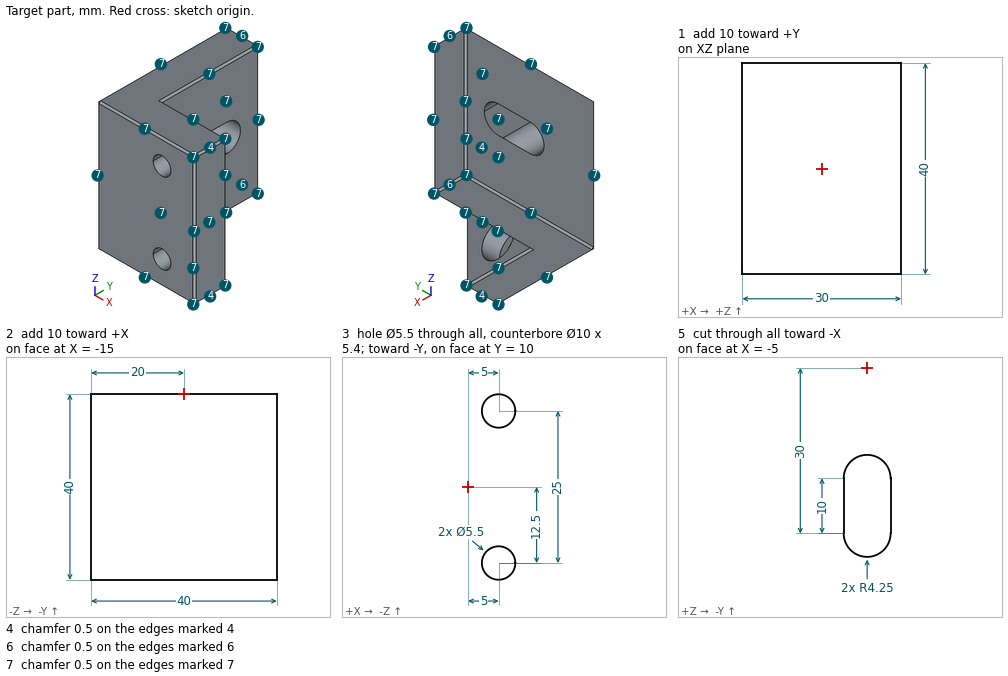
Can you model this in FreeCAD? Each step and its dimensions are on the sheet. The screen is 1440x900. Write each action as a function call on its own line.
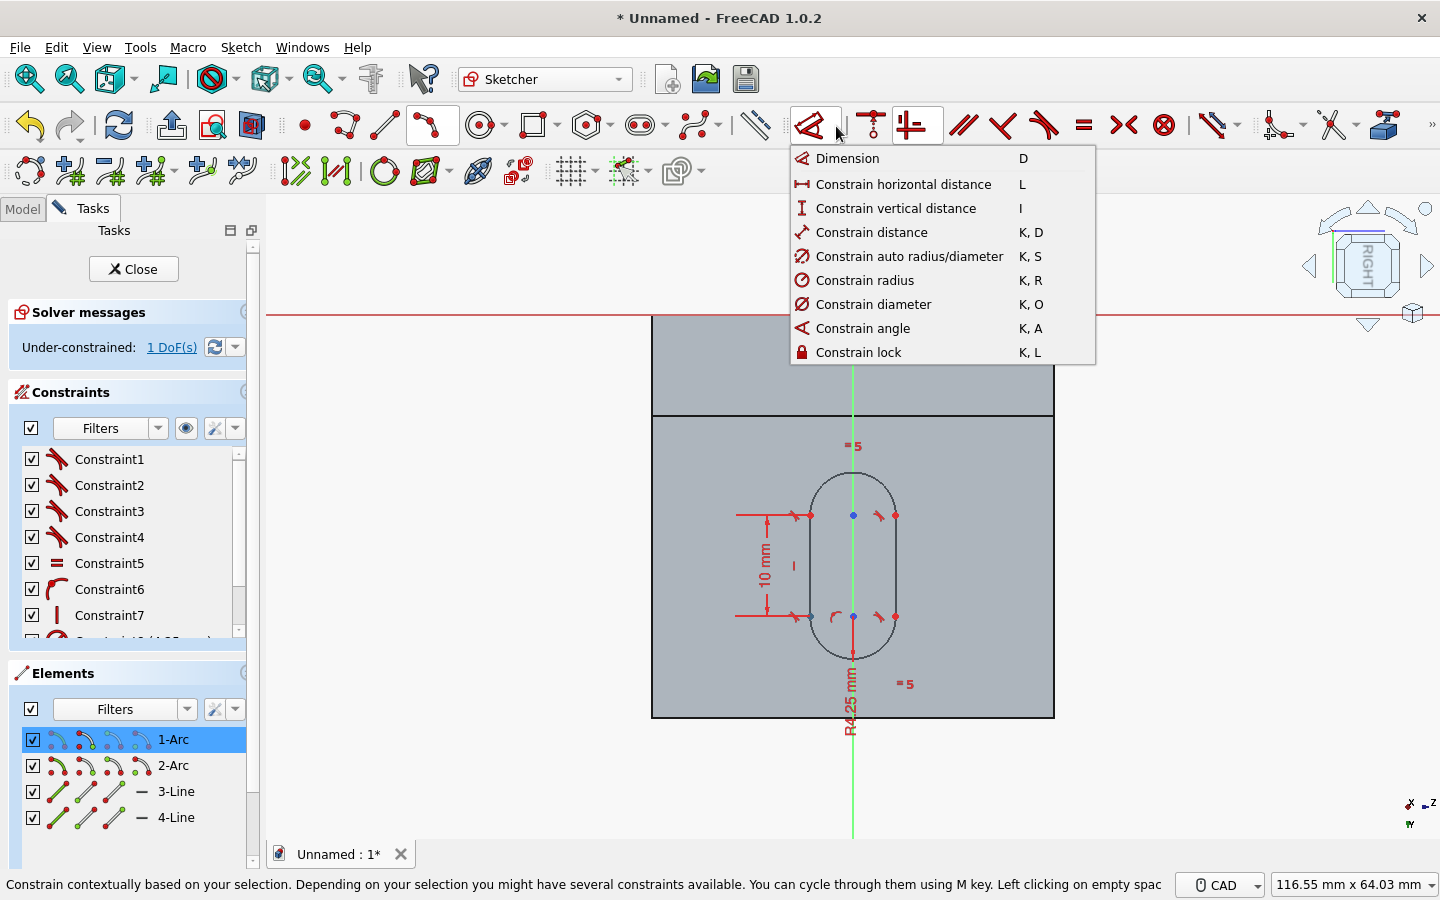
click(943, 208)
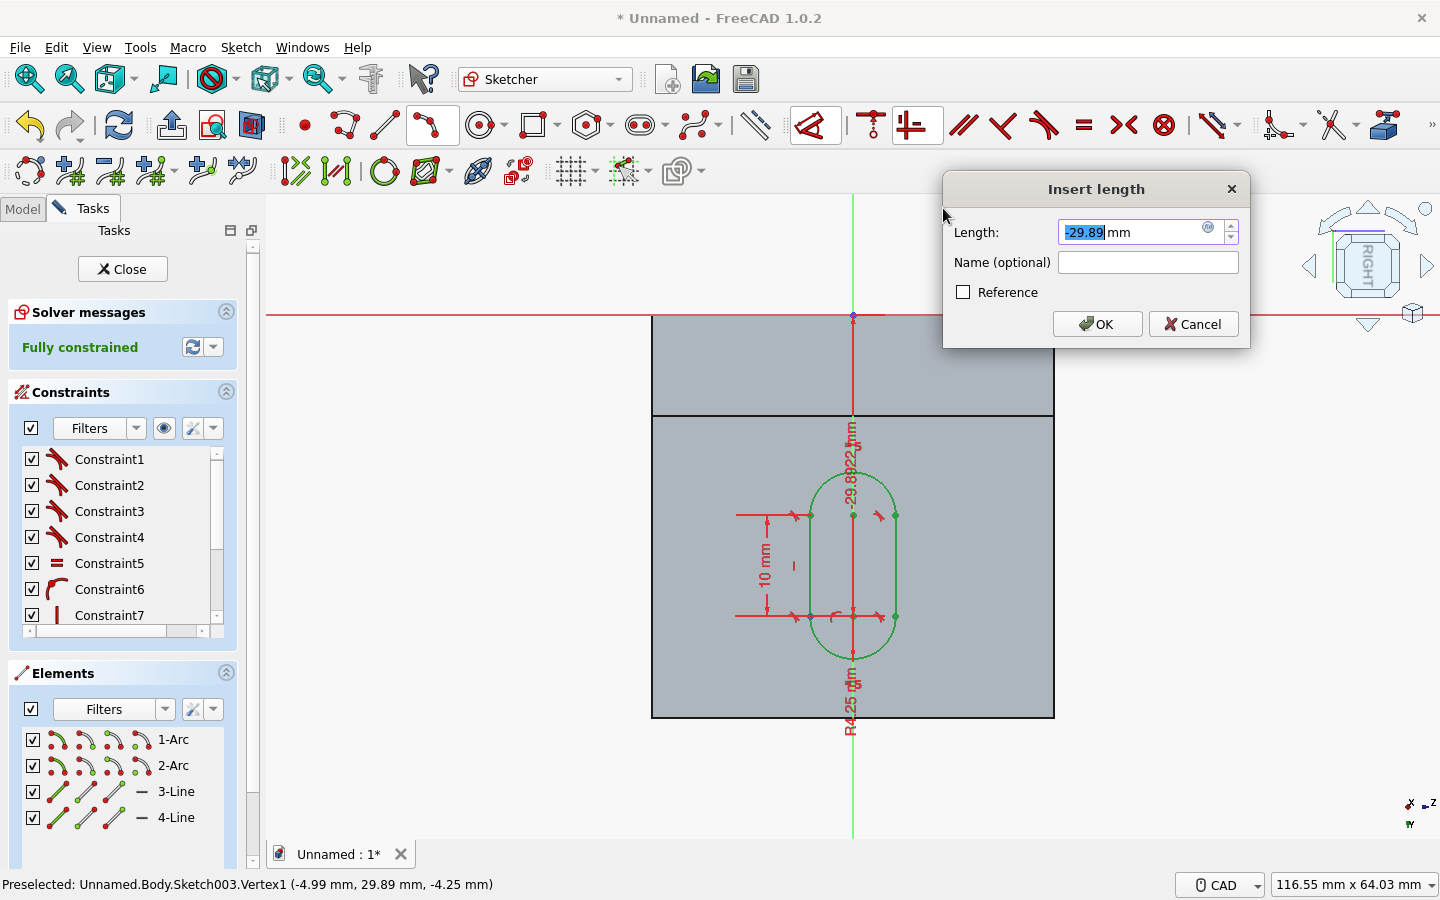
text(-30)
key(Return)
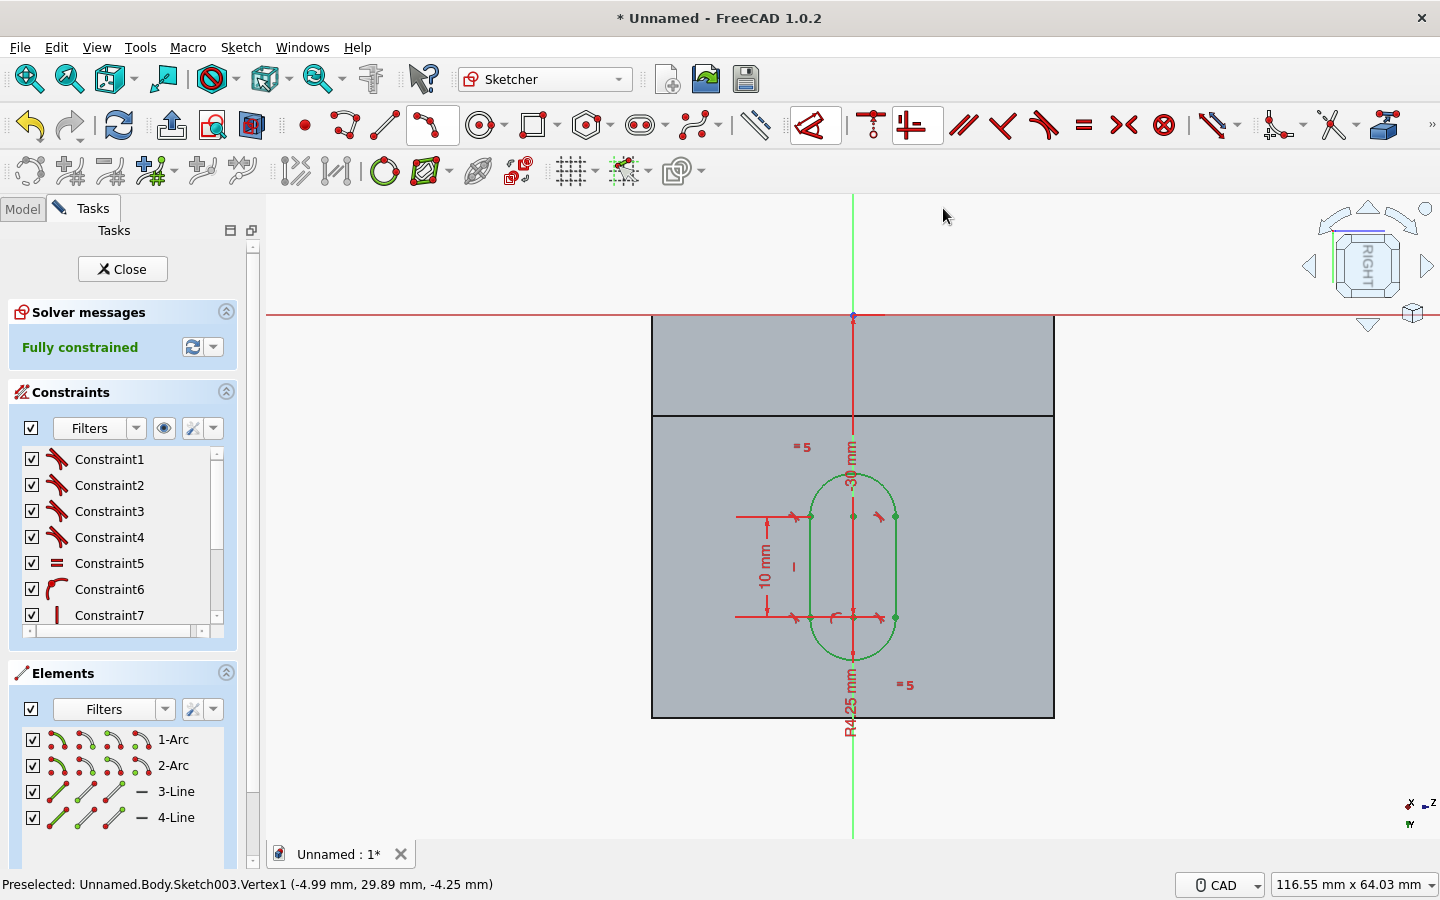
click(123, 269)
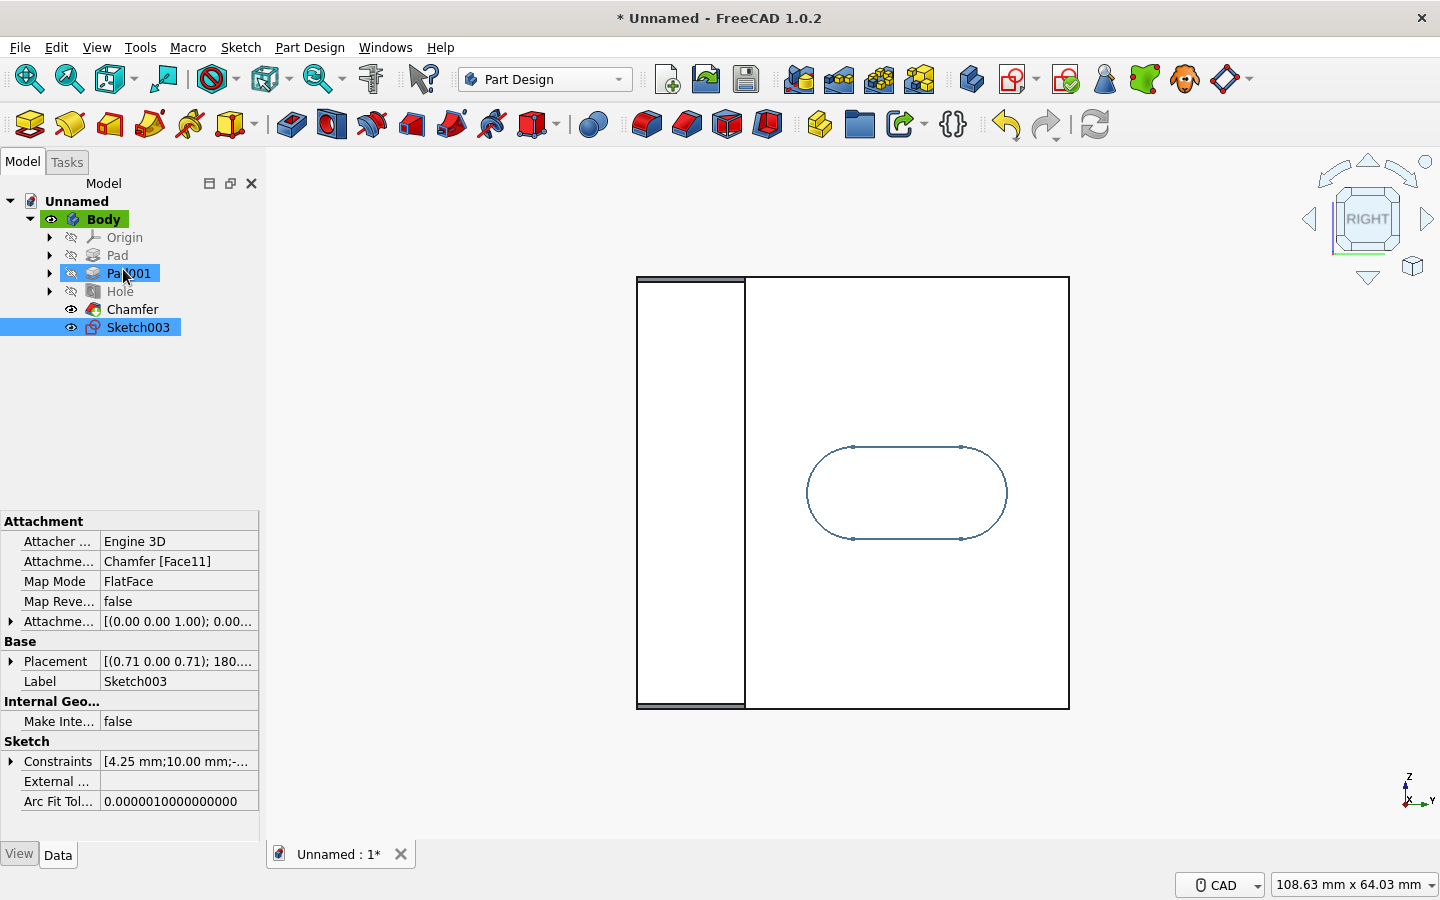
click(292, 124)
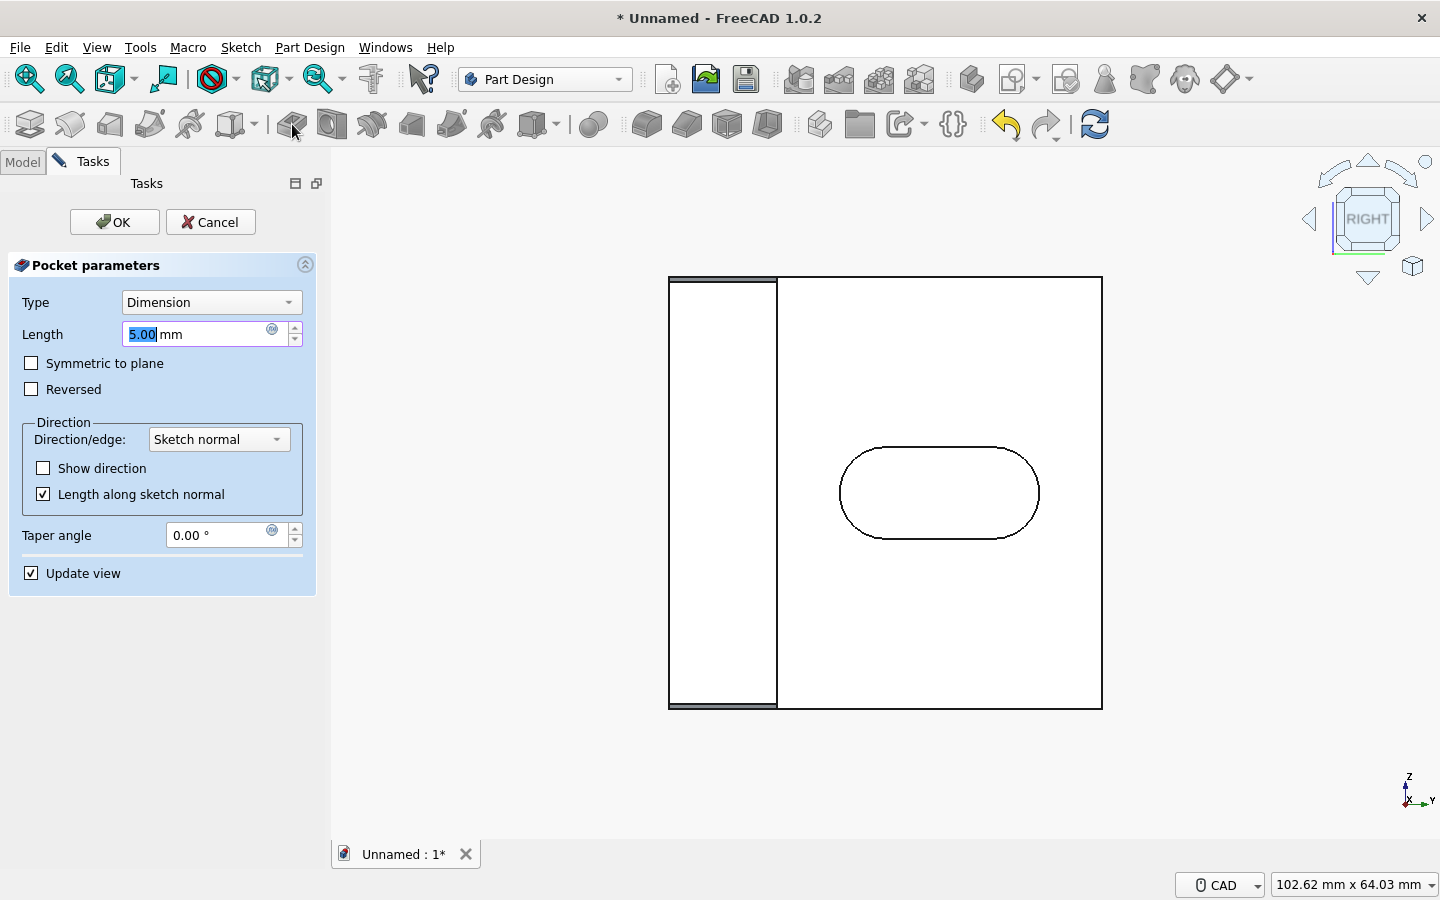
click(212, 302)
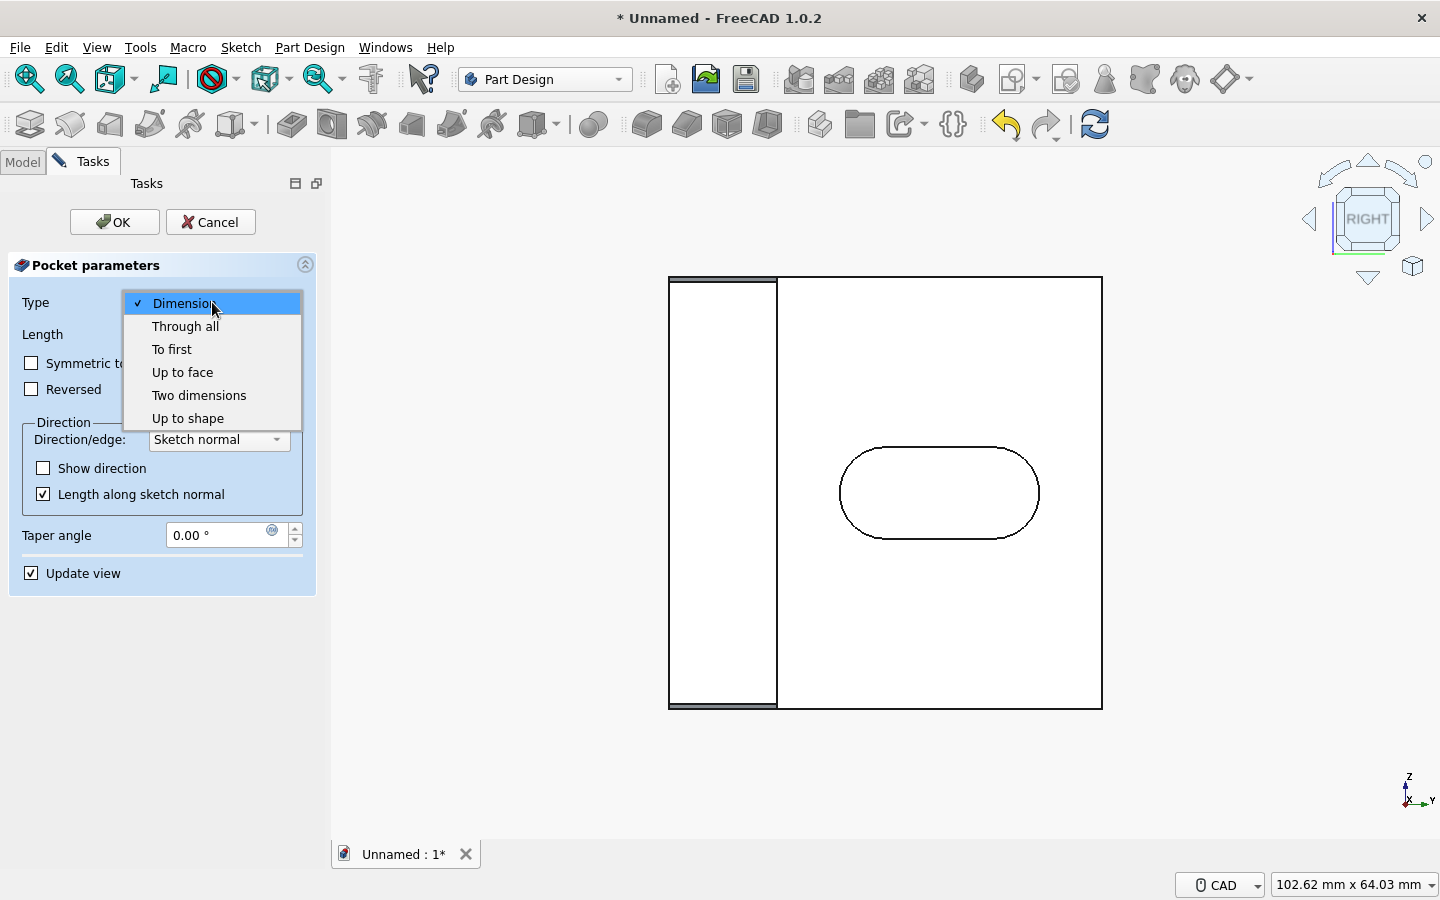
click(212, 326)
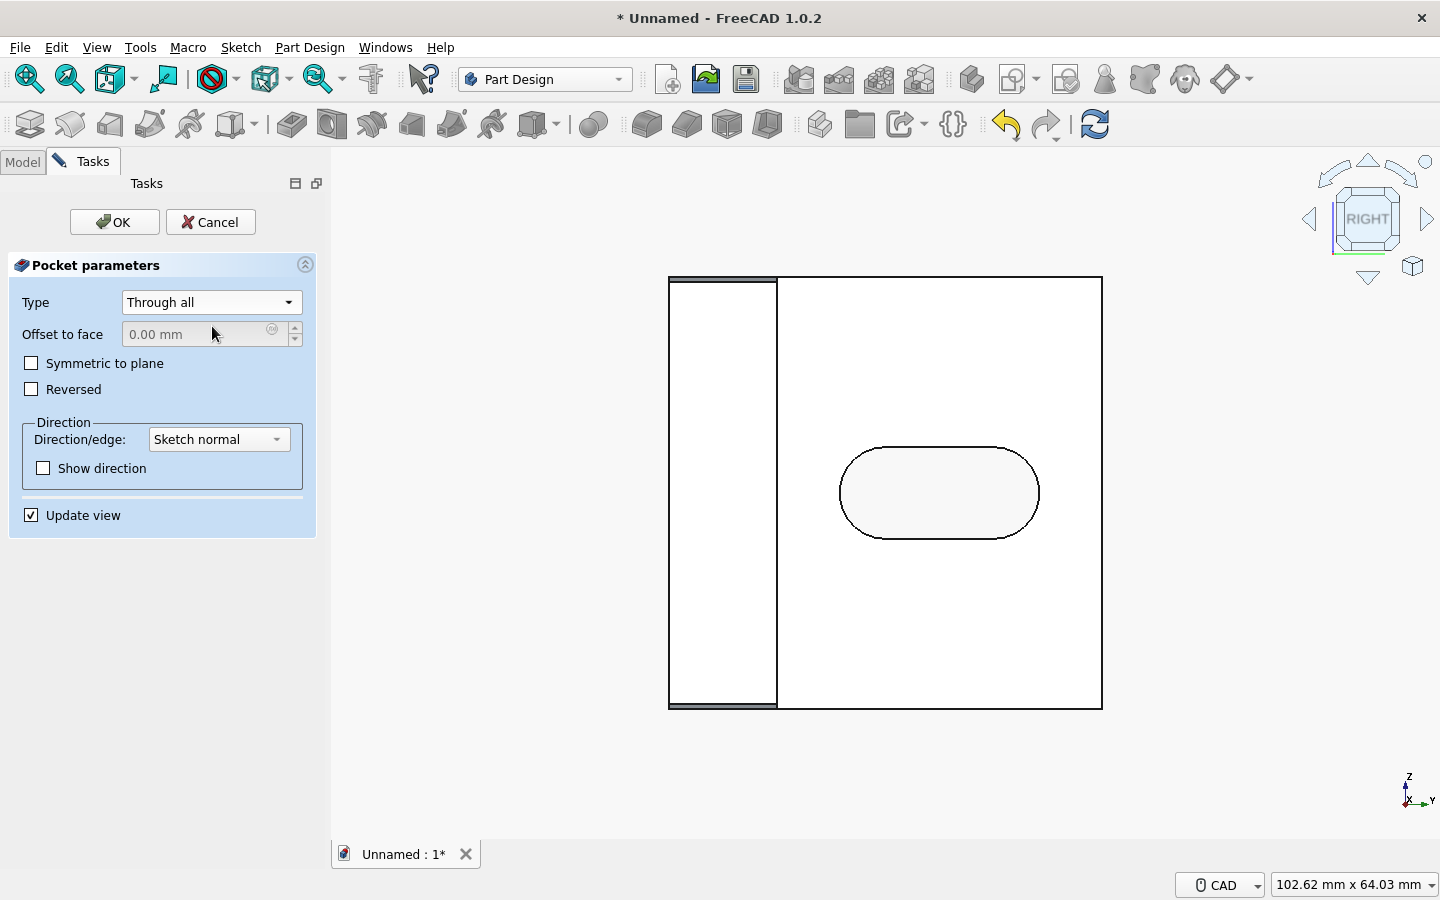
click(115, 222)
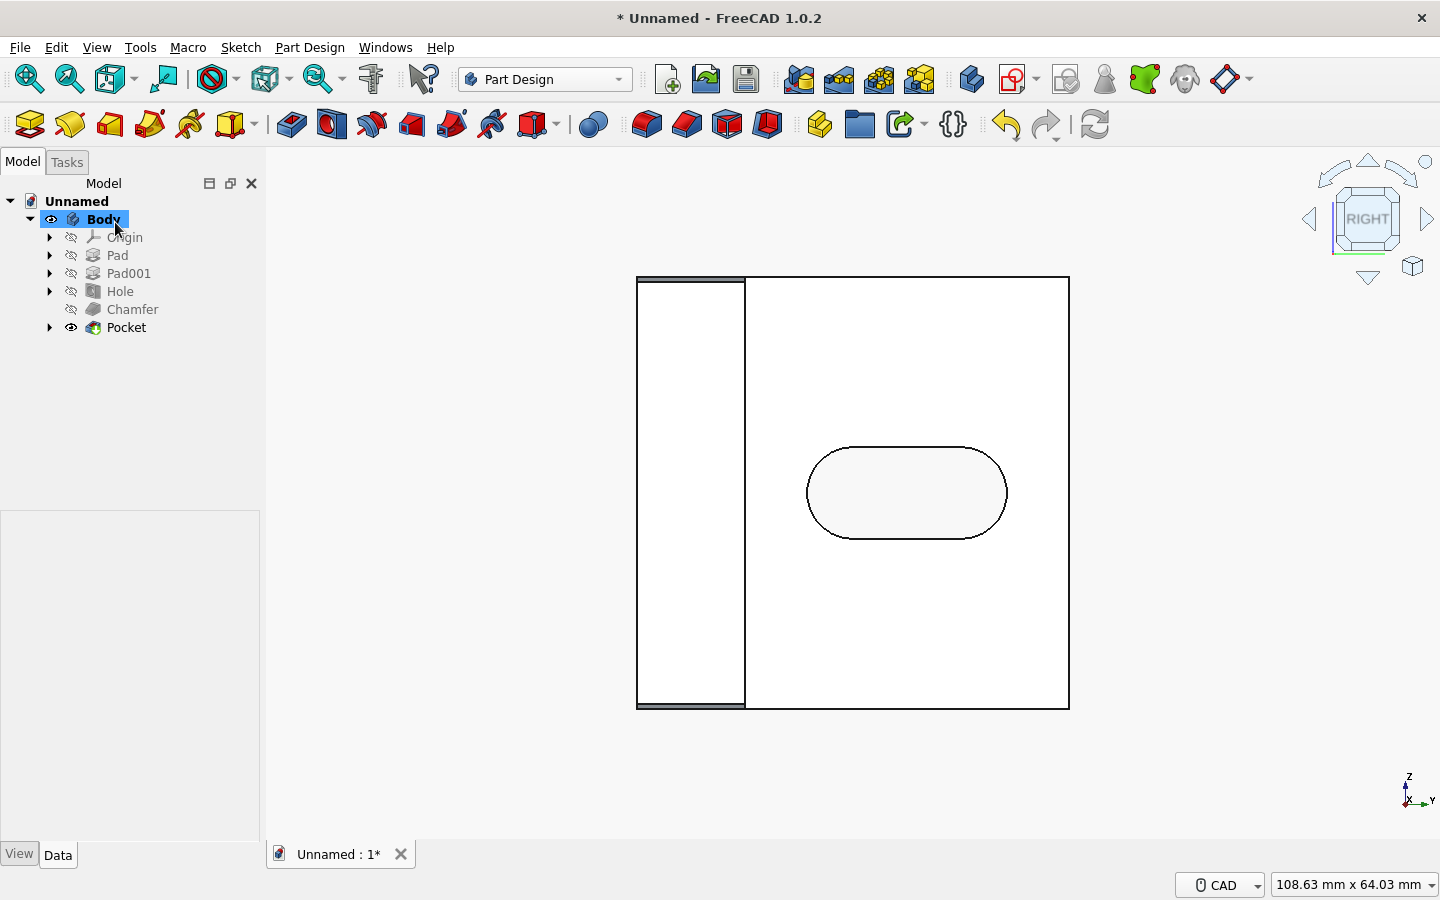
key(0)